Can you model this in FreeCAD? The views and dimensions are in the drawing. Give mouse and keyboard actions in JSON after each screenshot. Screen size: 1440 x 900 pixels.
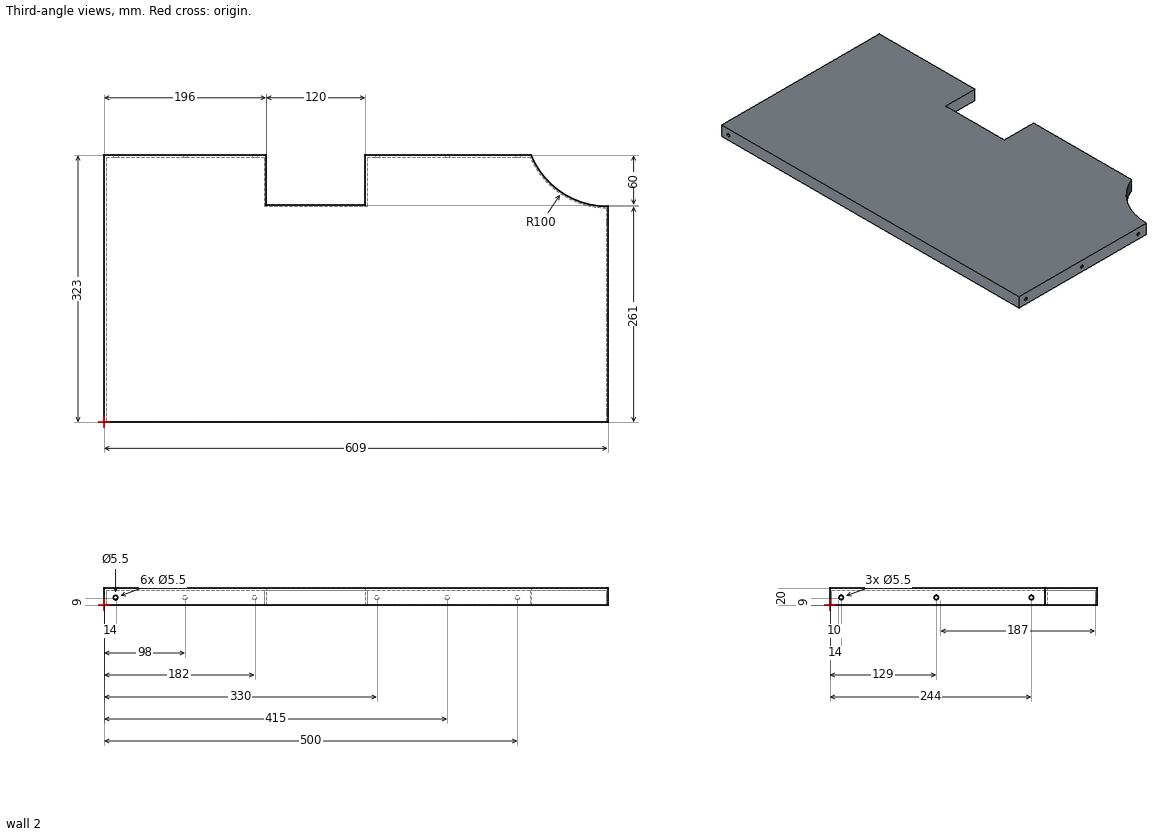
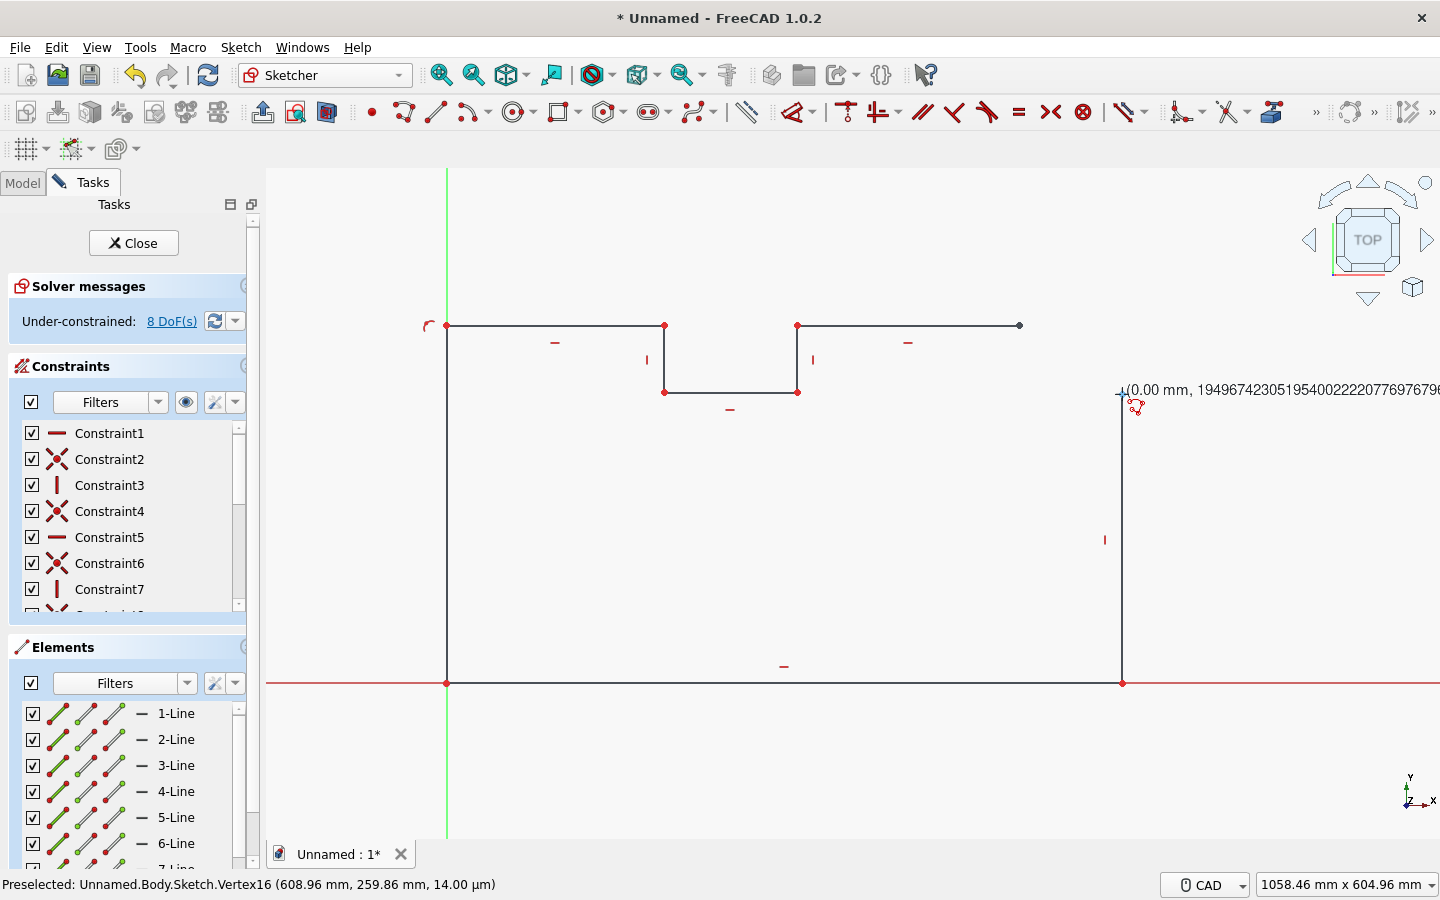
{"action": "key", "text": "g 3 a"}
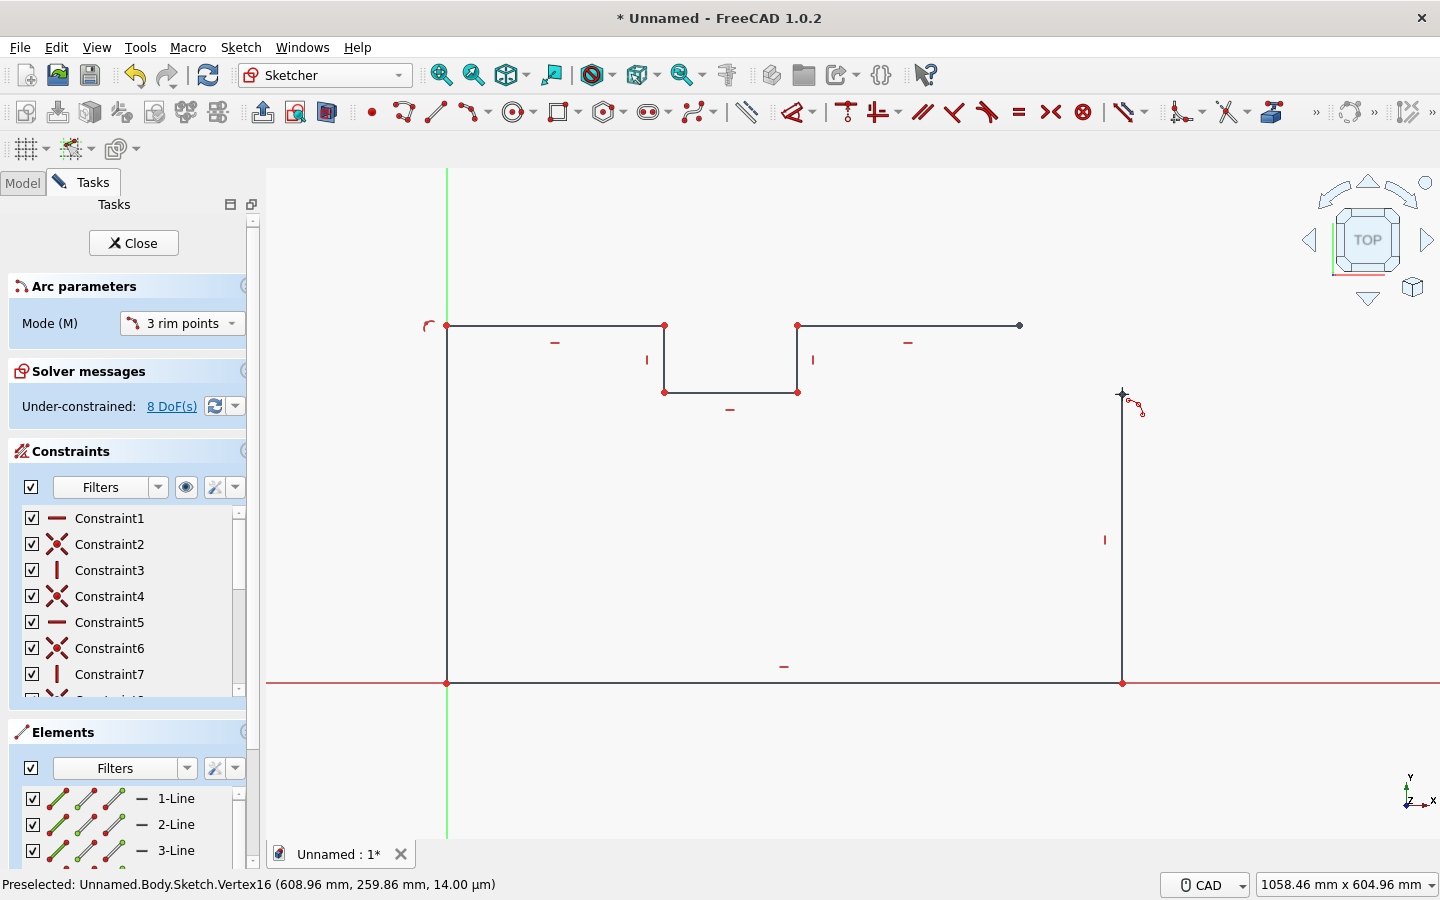
{"action": "left_click", "coordinate": [1122, 395]}
{"action": "left_click", "coordinate": [1019, 326]}
{"action": "left_click", "coordinate": [1060, 375]}
{"action": "key", "text": "Escape"}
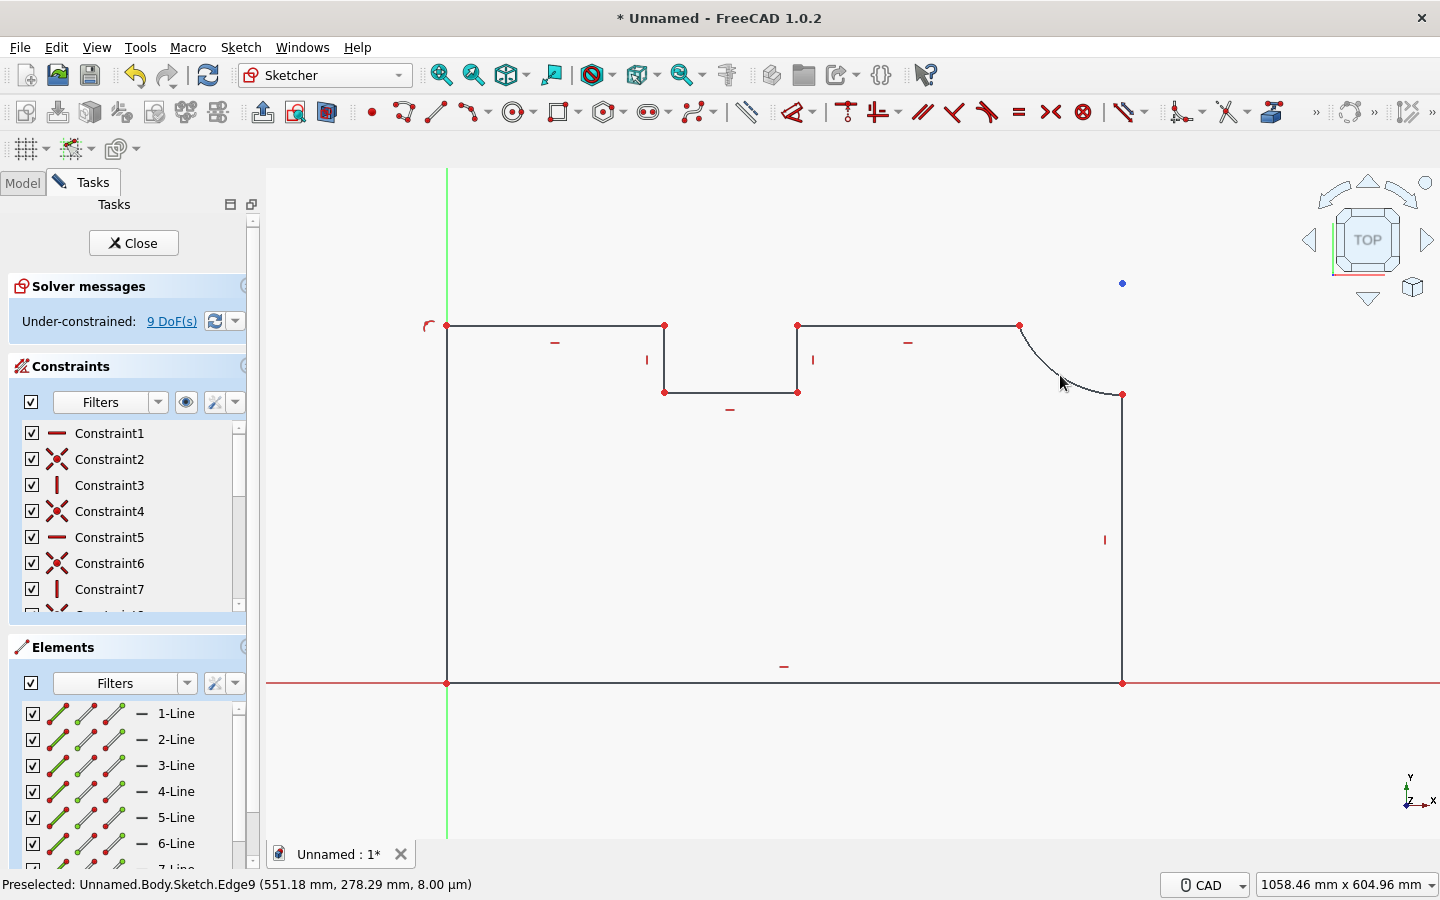
{"action": "left_click", "coordinate": [792, 112]}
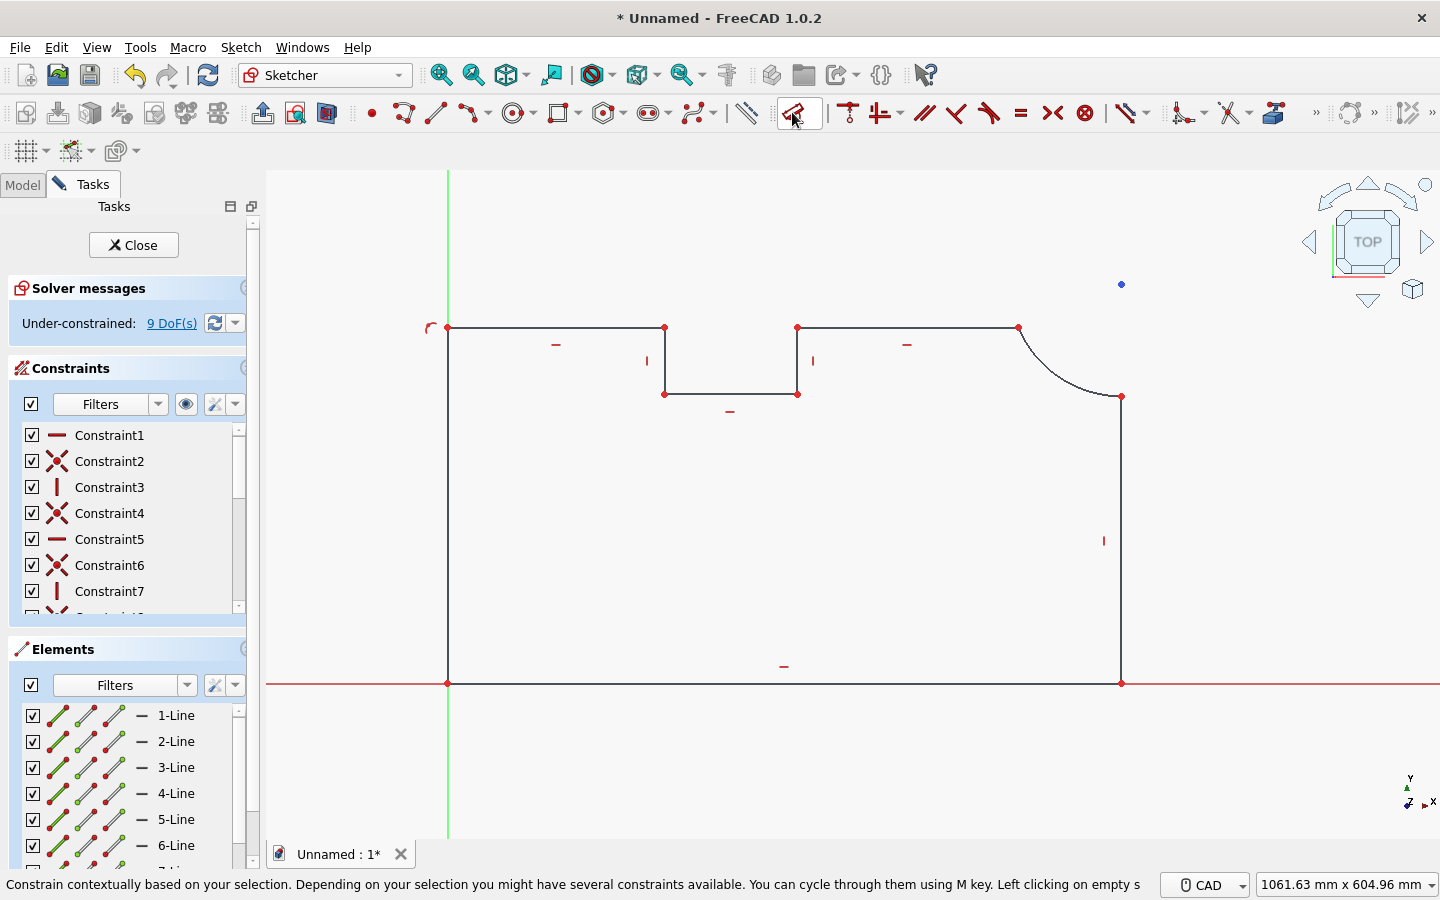
{"action": "left_click", "coordinate": [1040, 360]}
{"action": "left_click", "coordinate": [1016, 382]}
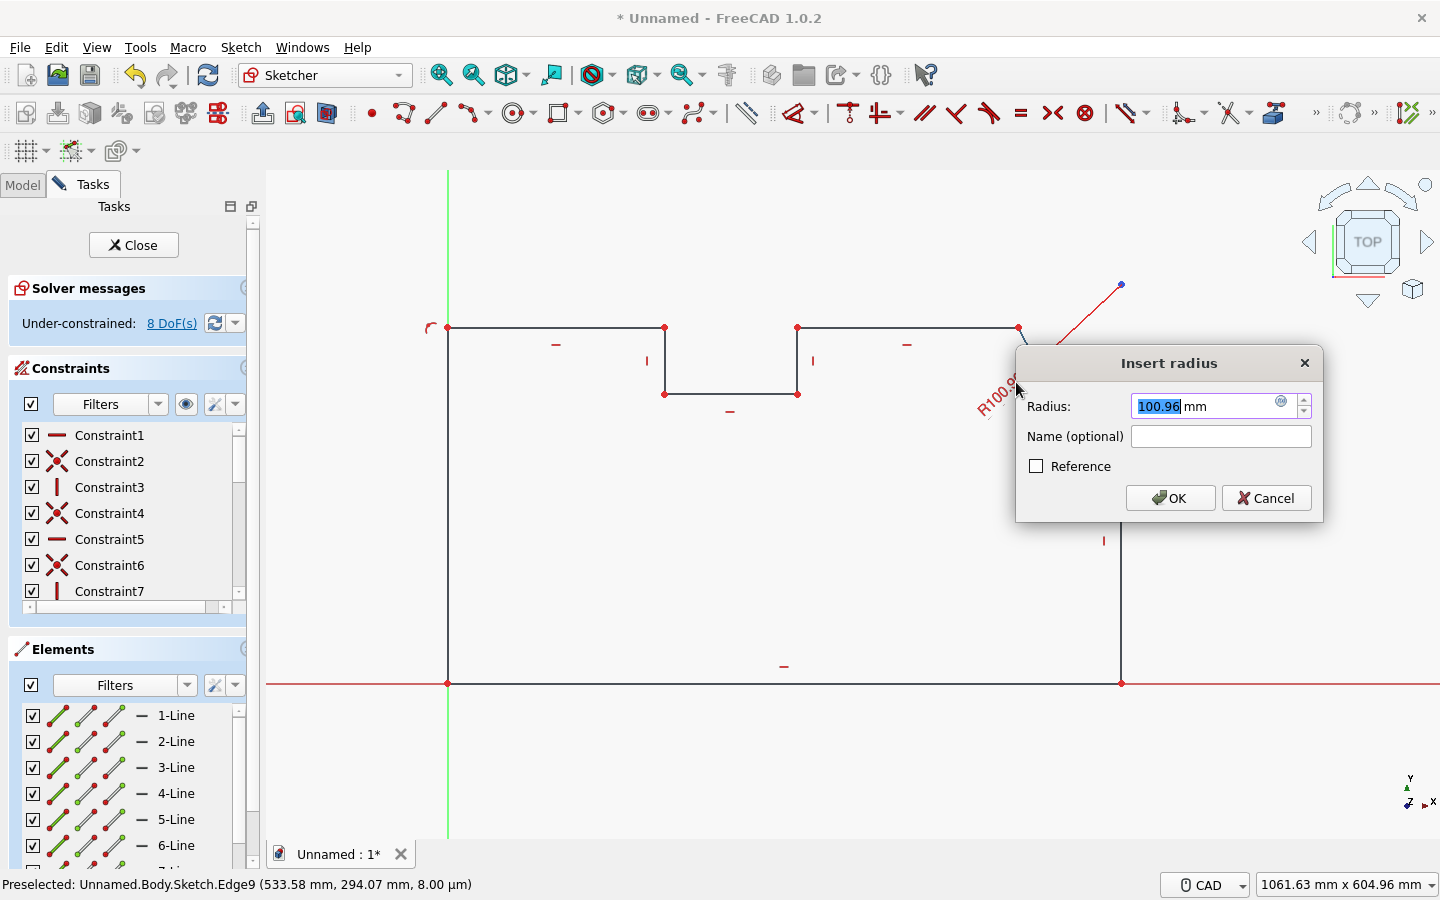
{"action": "type", "text": "100"}
{"action": "key", "text": "Return"}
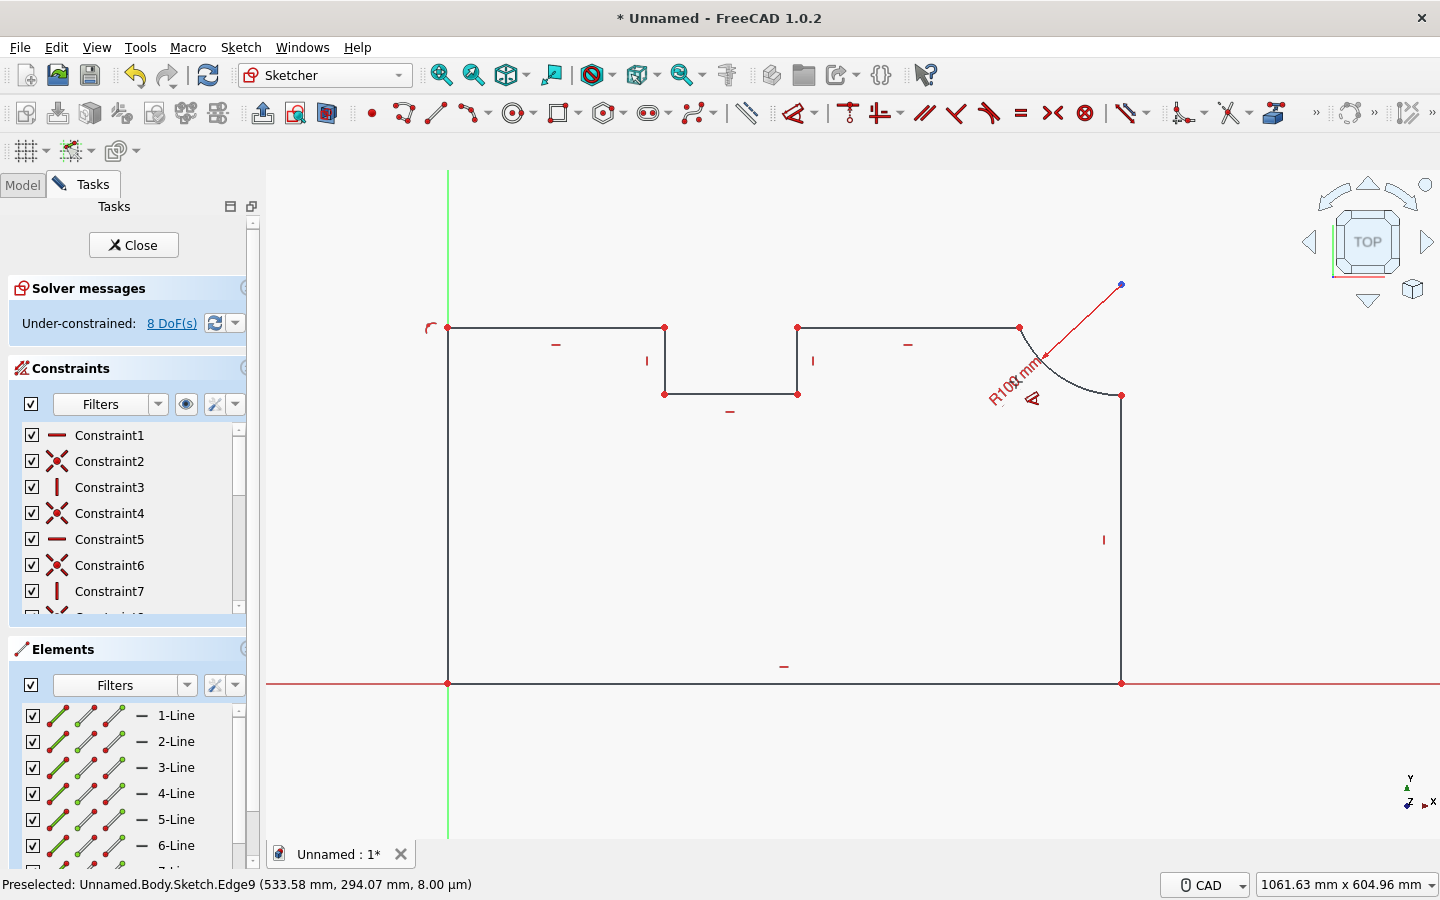
{"action": "left_click", "coordinate": [797, 348]}
{"action": "left_click", "coordinate": [831, 361]}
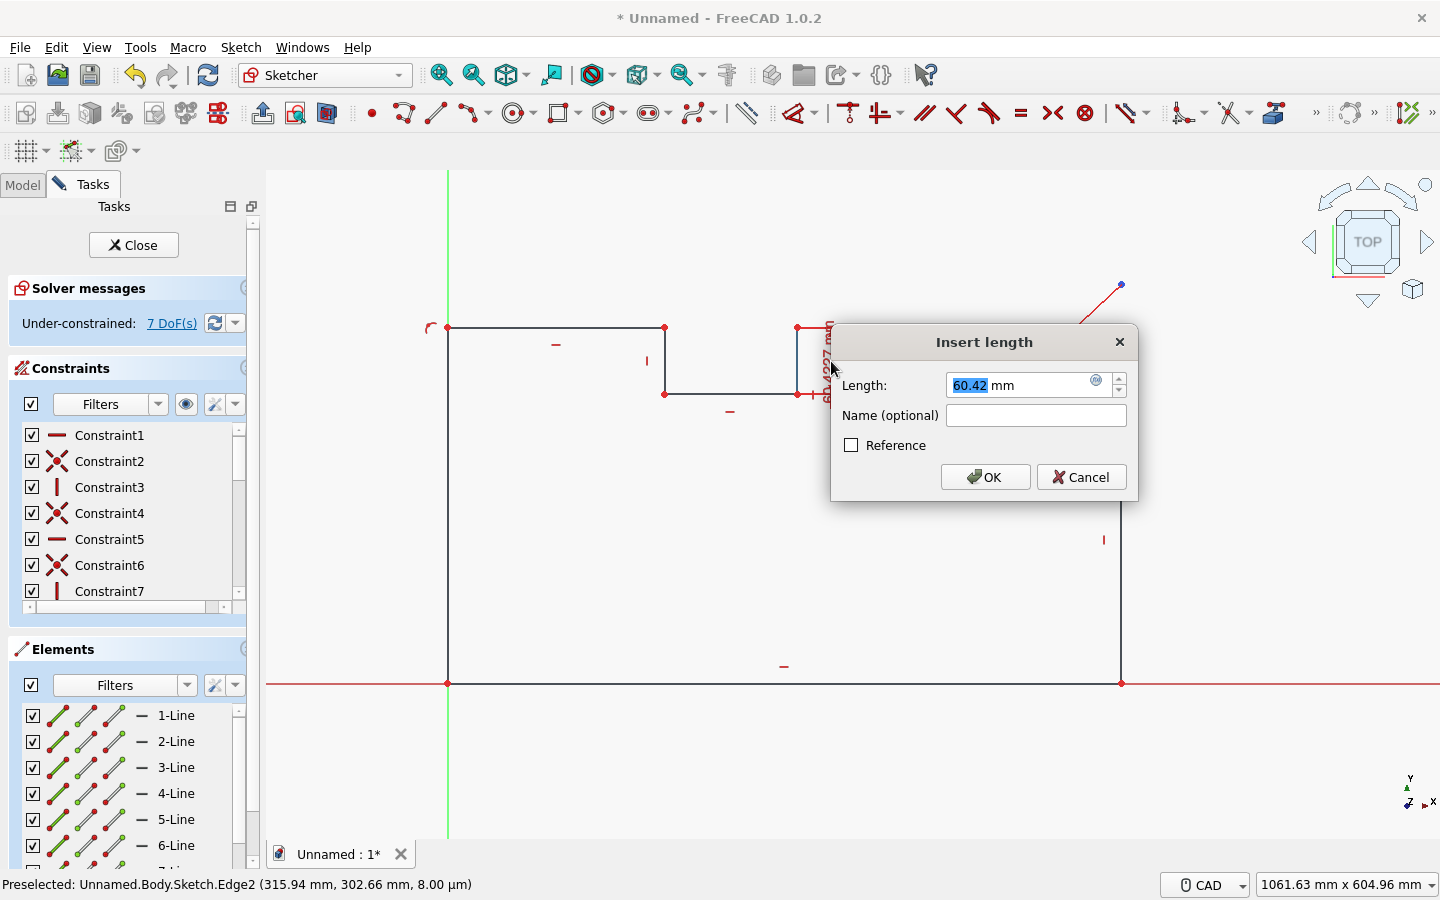
{"action": "type", "text": "60"}
{"action": "key", "text": "Return"}